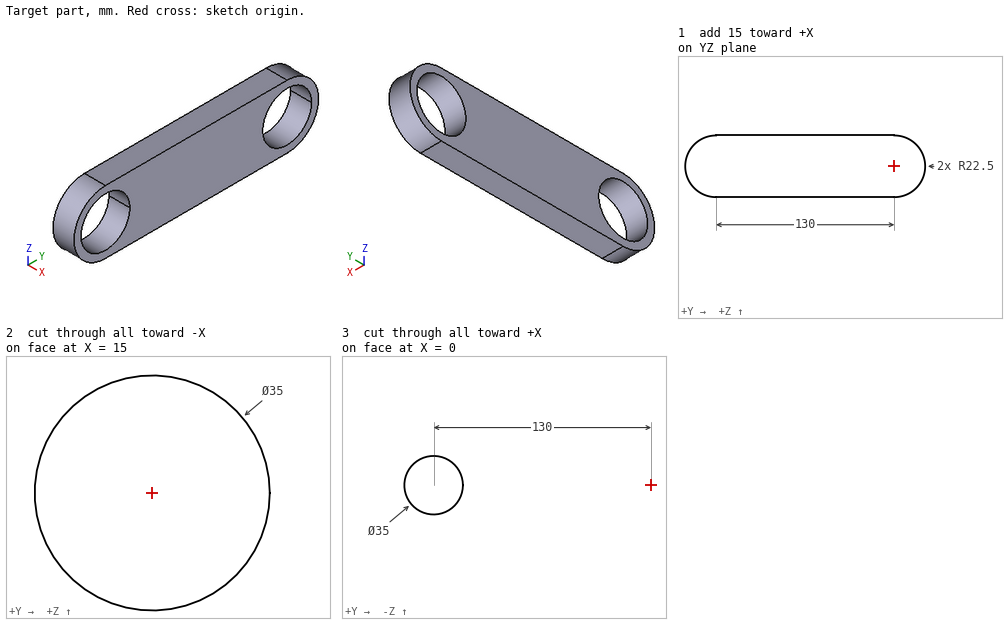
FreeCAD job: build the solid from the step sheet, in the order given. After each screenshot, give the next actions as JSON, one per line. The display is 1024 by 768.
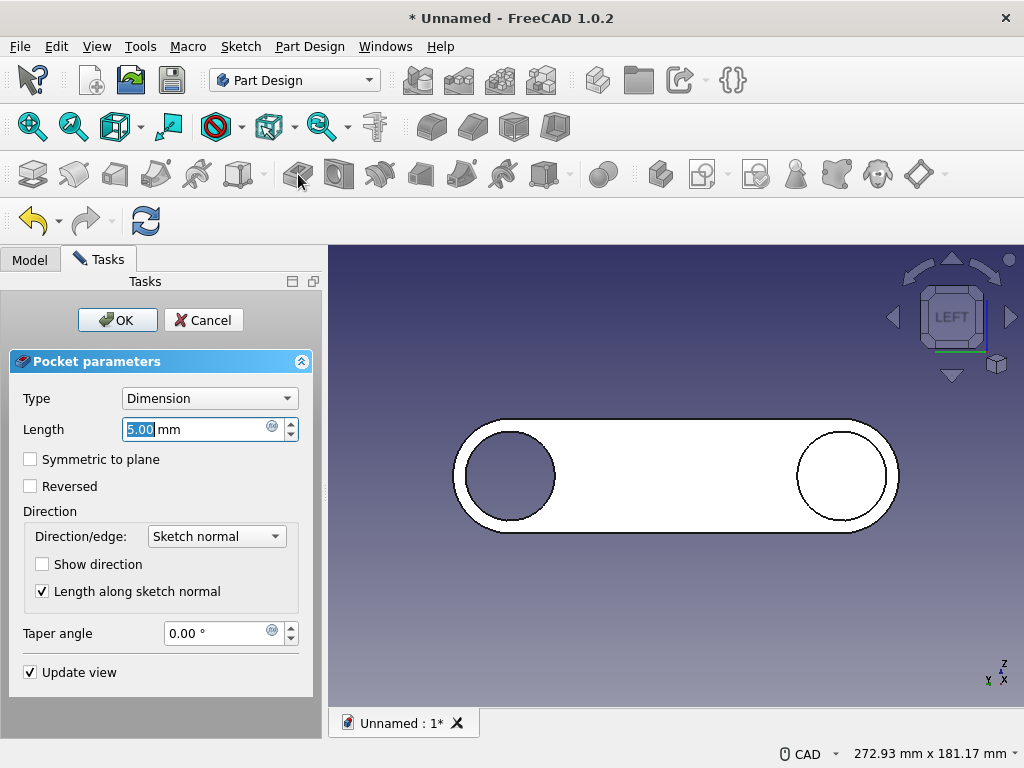
{"action": "left_click", "coordinate": [210, 398]}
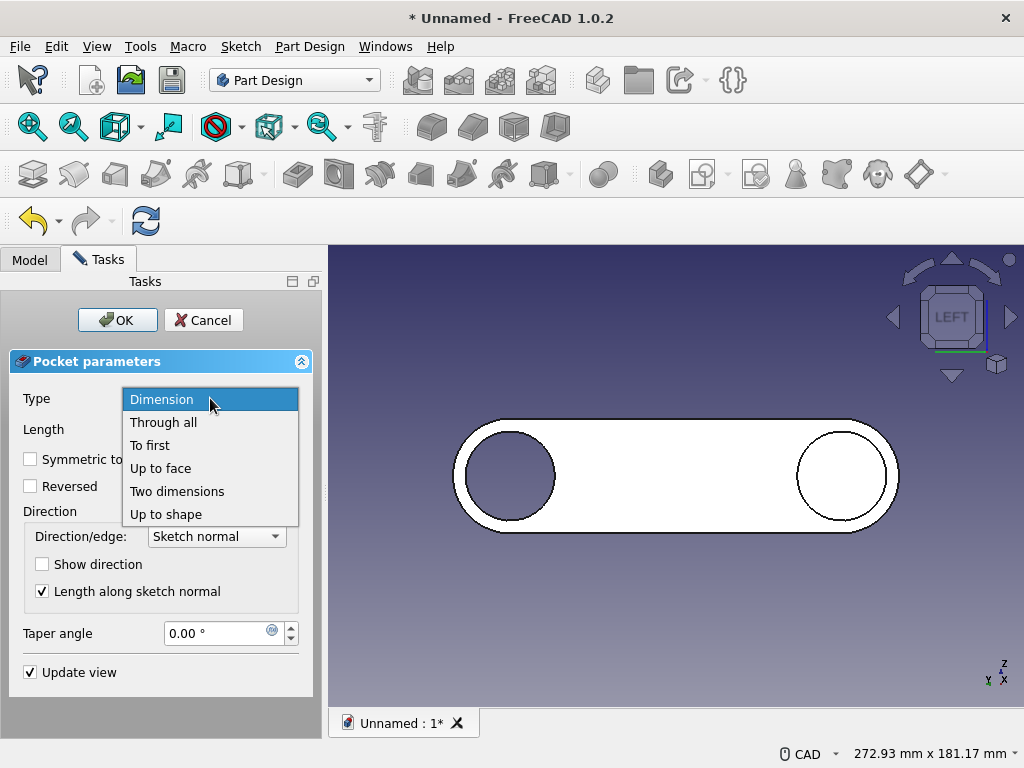
{"action": "left_click", "coordinate": [208, 422]}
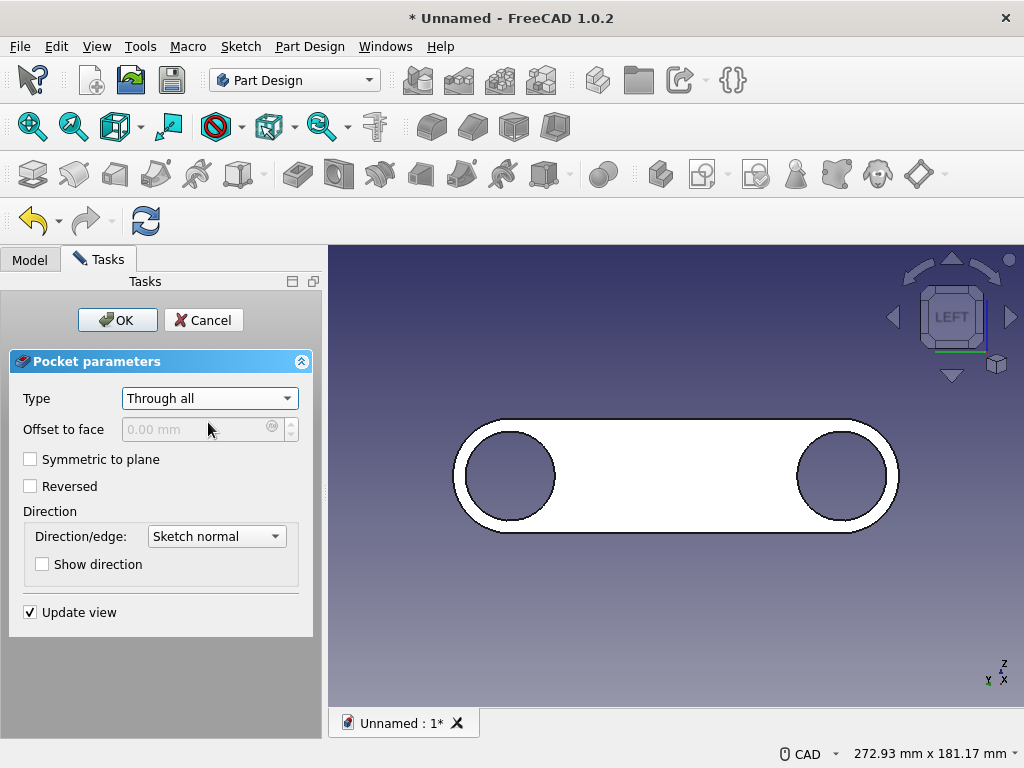
{"action": "left_click", "coordinate": [118, 320]}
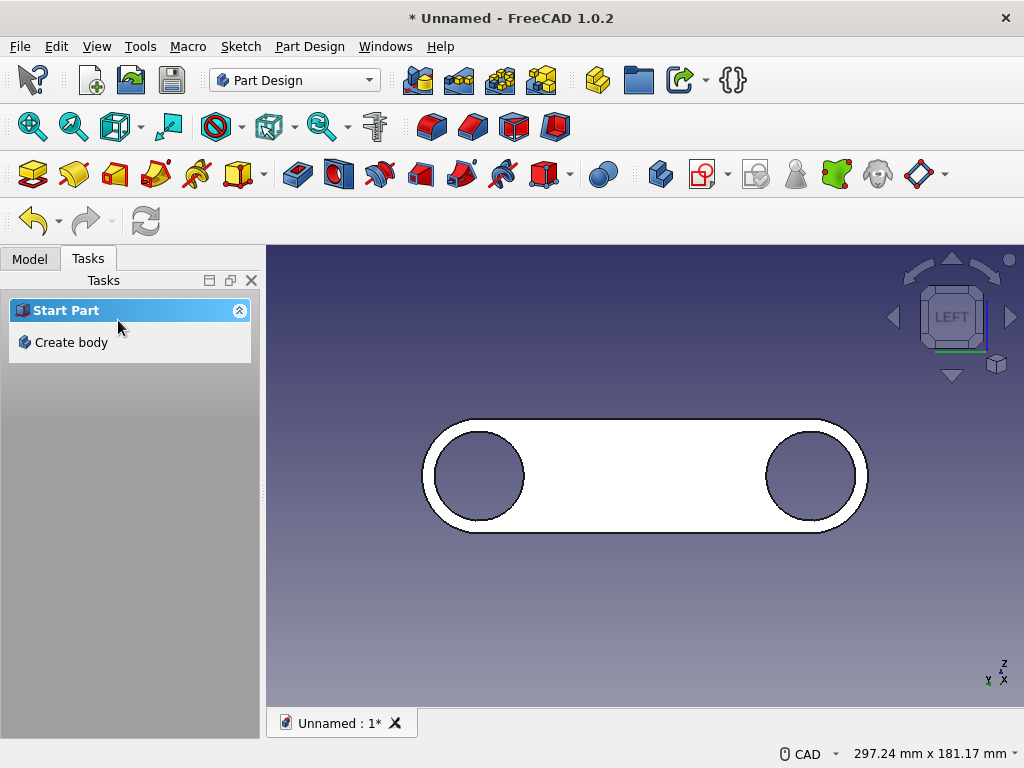
{"action": "key", "text": "0"}